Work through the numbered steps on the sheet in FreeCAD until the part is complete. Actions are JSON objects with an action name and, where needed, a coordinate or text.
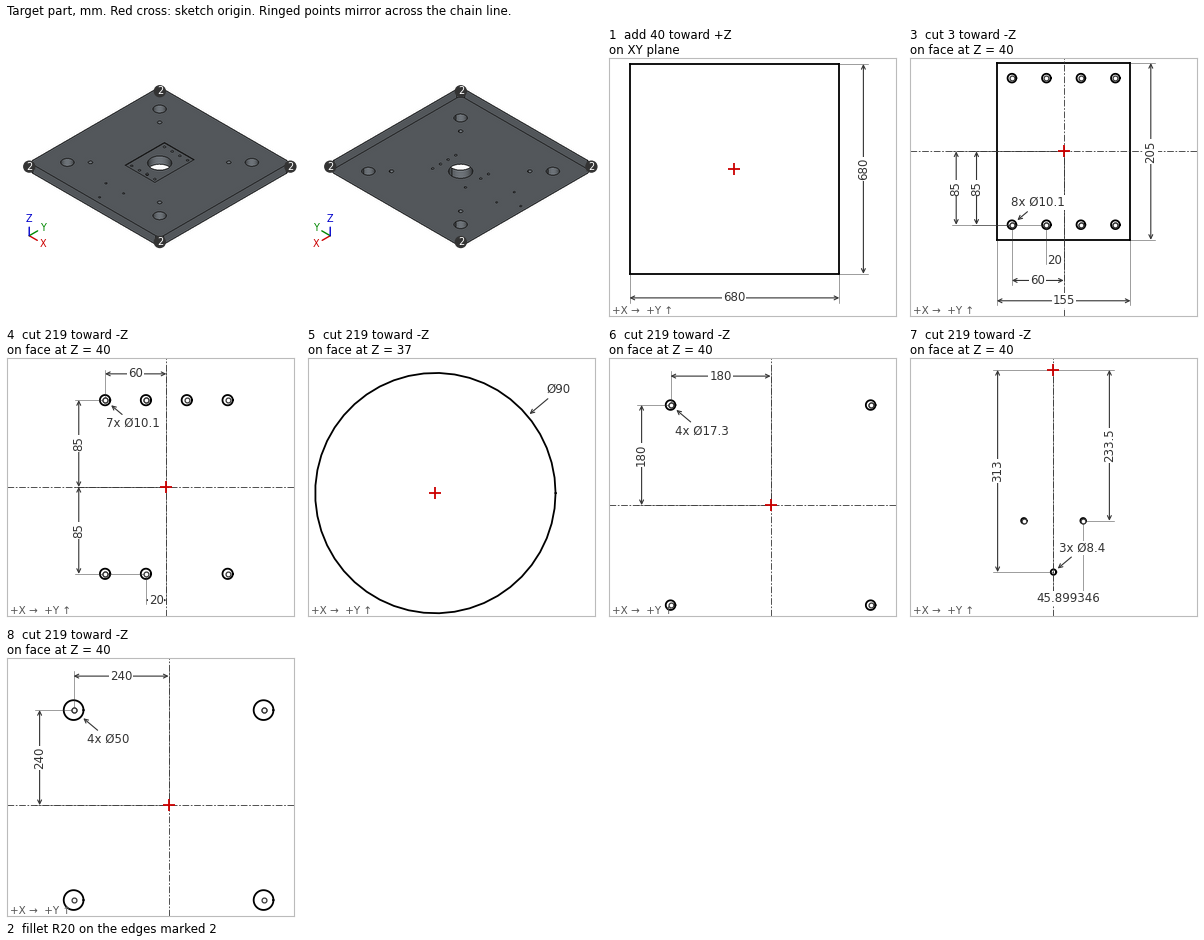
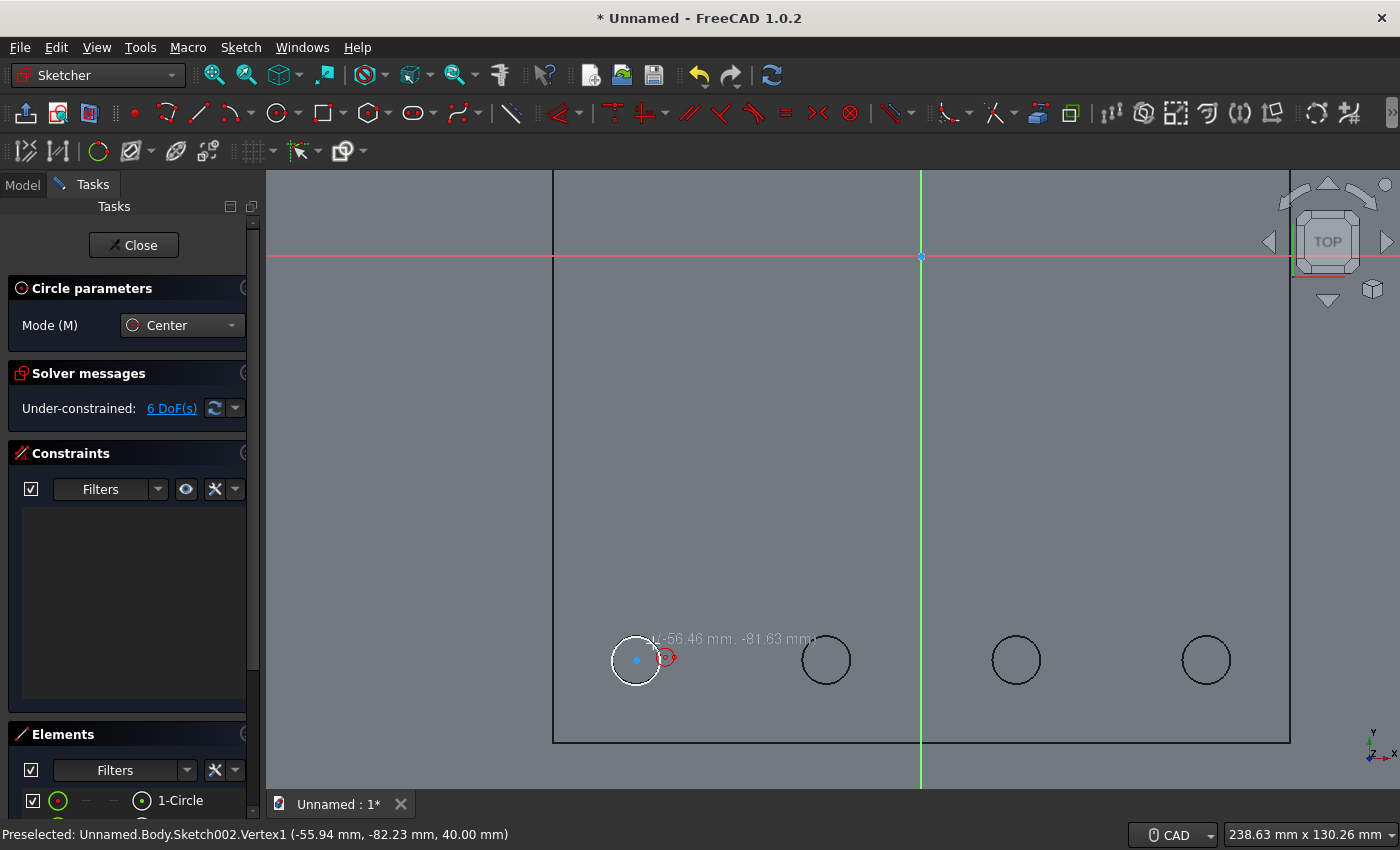
{"action": "left_click", "coordinate": [826, 660]}
{"action": "left_click", "coordinate": [843, 643]}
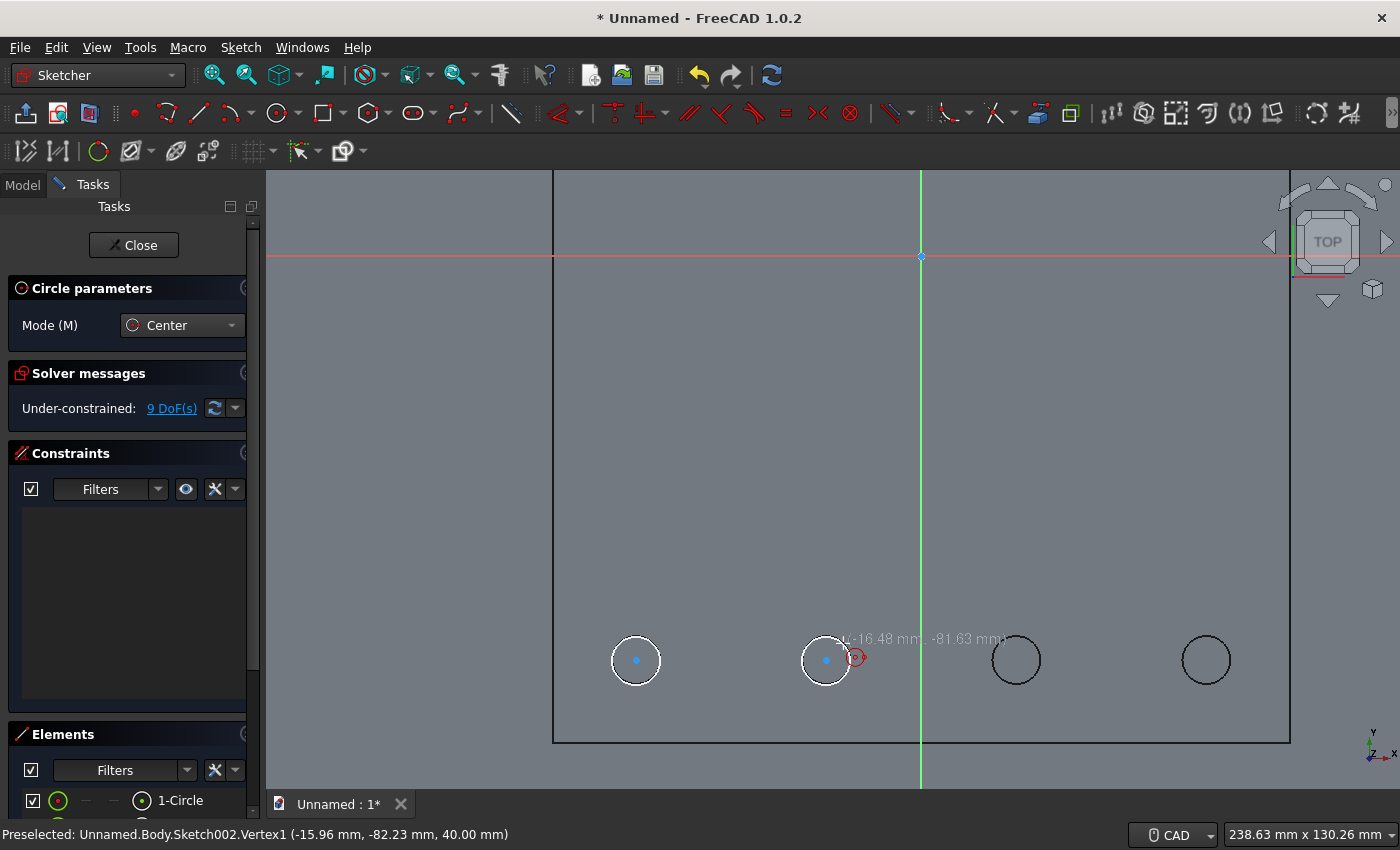
{"action": "left_click", "coordinate": [1206, 660]}
{"action": "left_click", "coordinate": [1223, 643]}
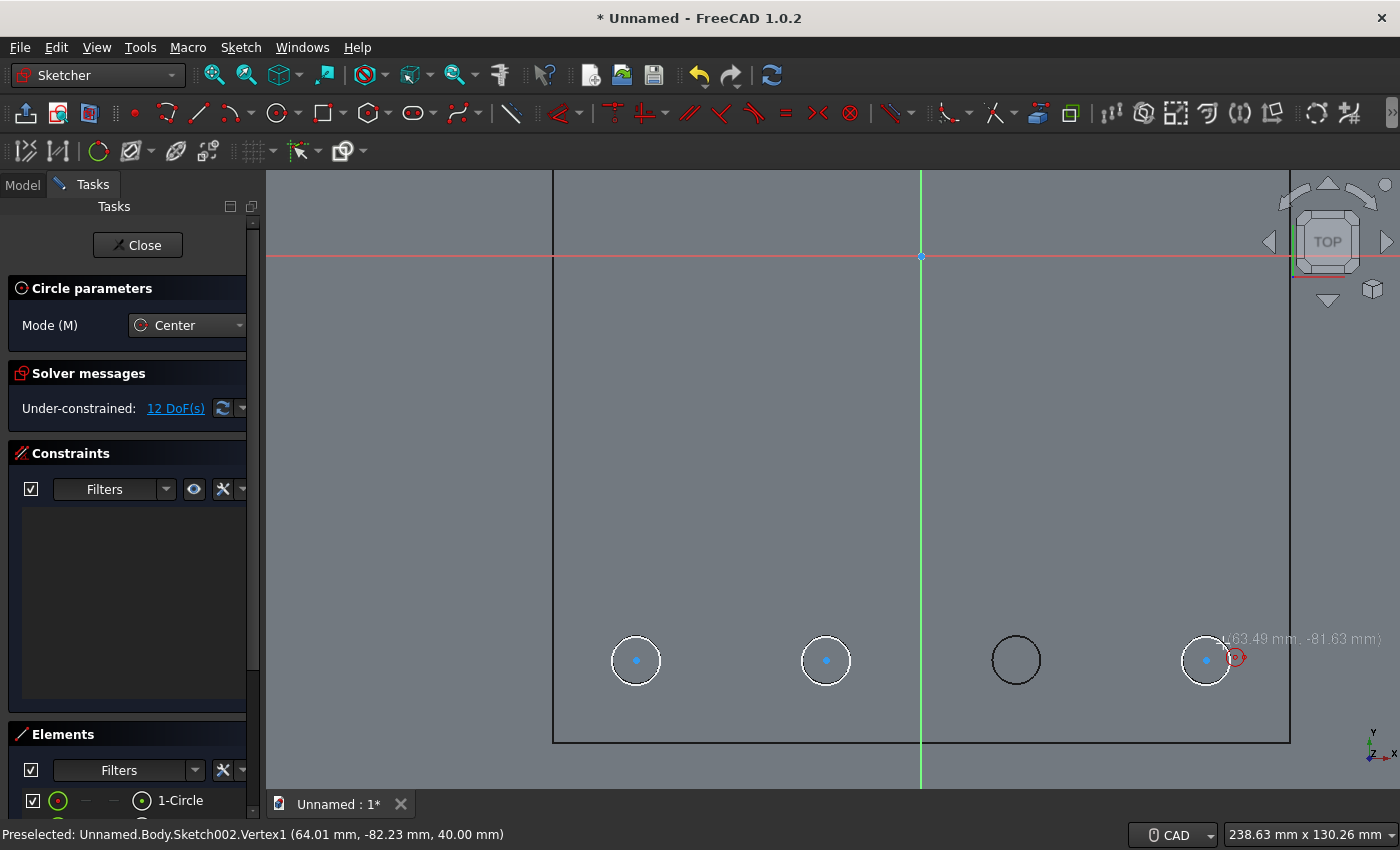
{"action": "scroll", "coordinate": [637, 662], "scroll_direction": "down", "scroll_amount": 4}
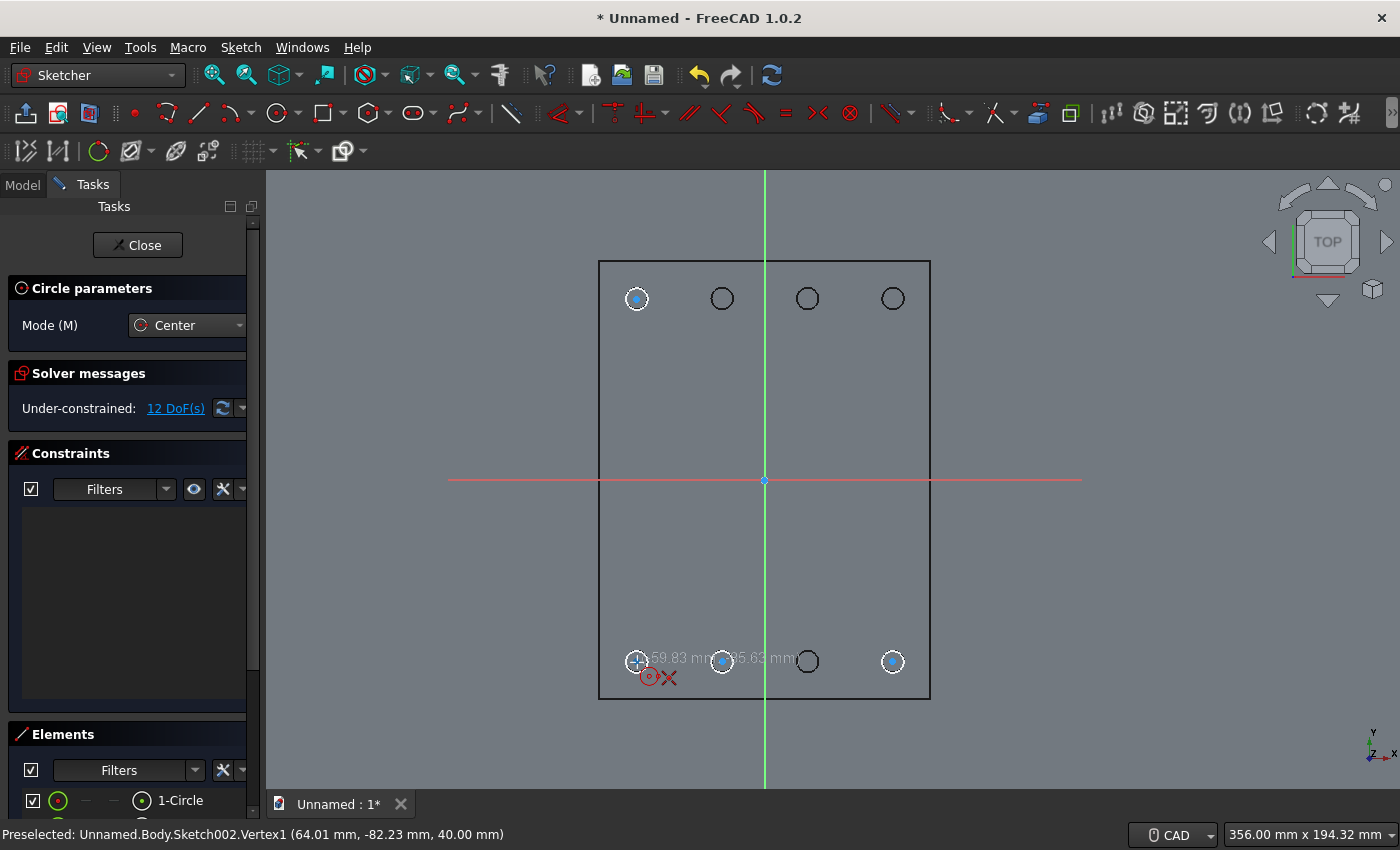
{"action": "scroll", "coordinate": [893, 299], "scroll_direction": "up", "scroll_amount": 4}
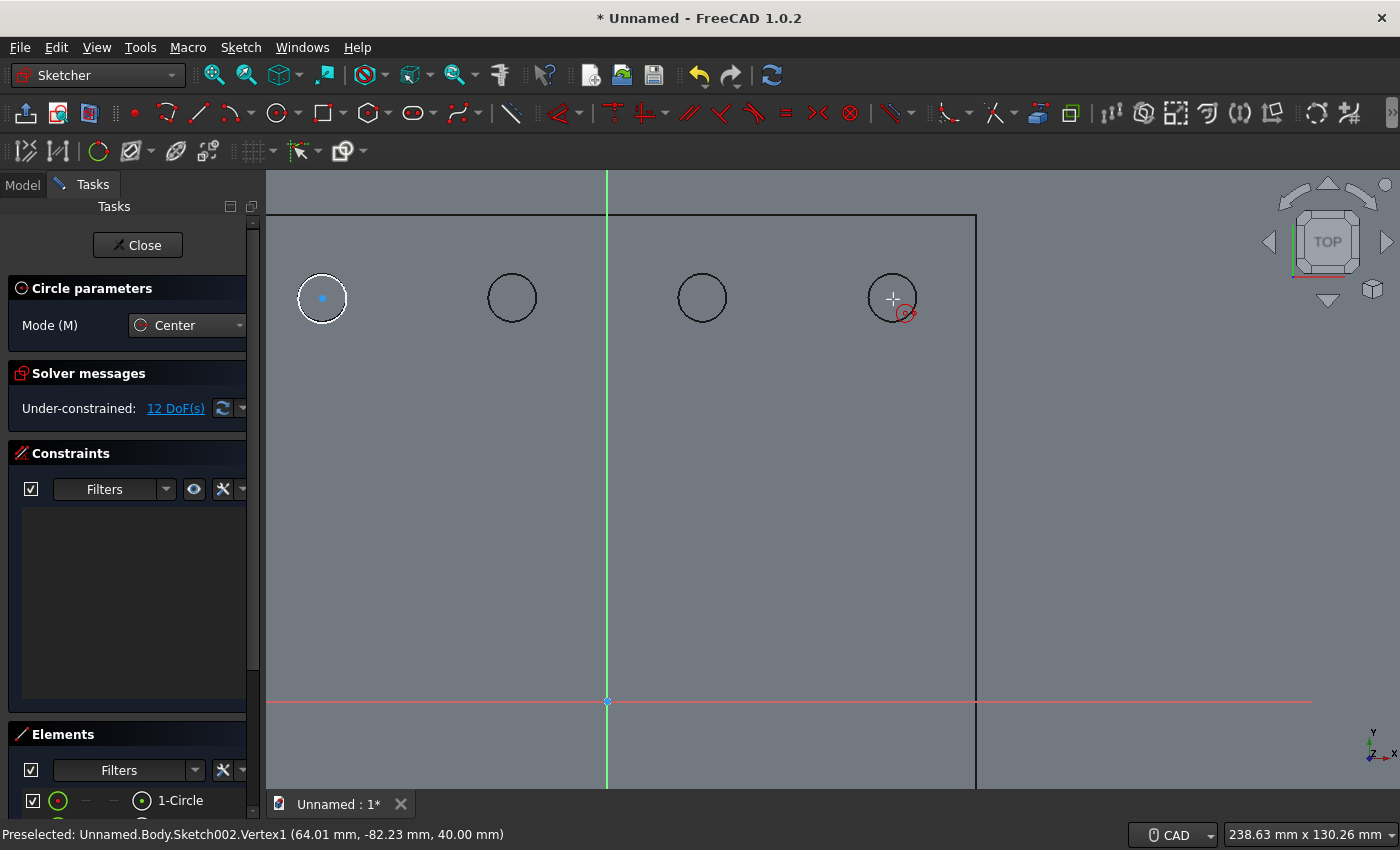
{"action": "left_click", "coordinate": [892, 298]}
{"action": "left_click", "coordinate": [909, 281]}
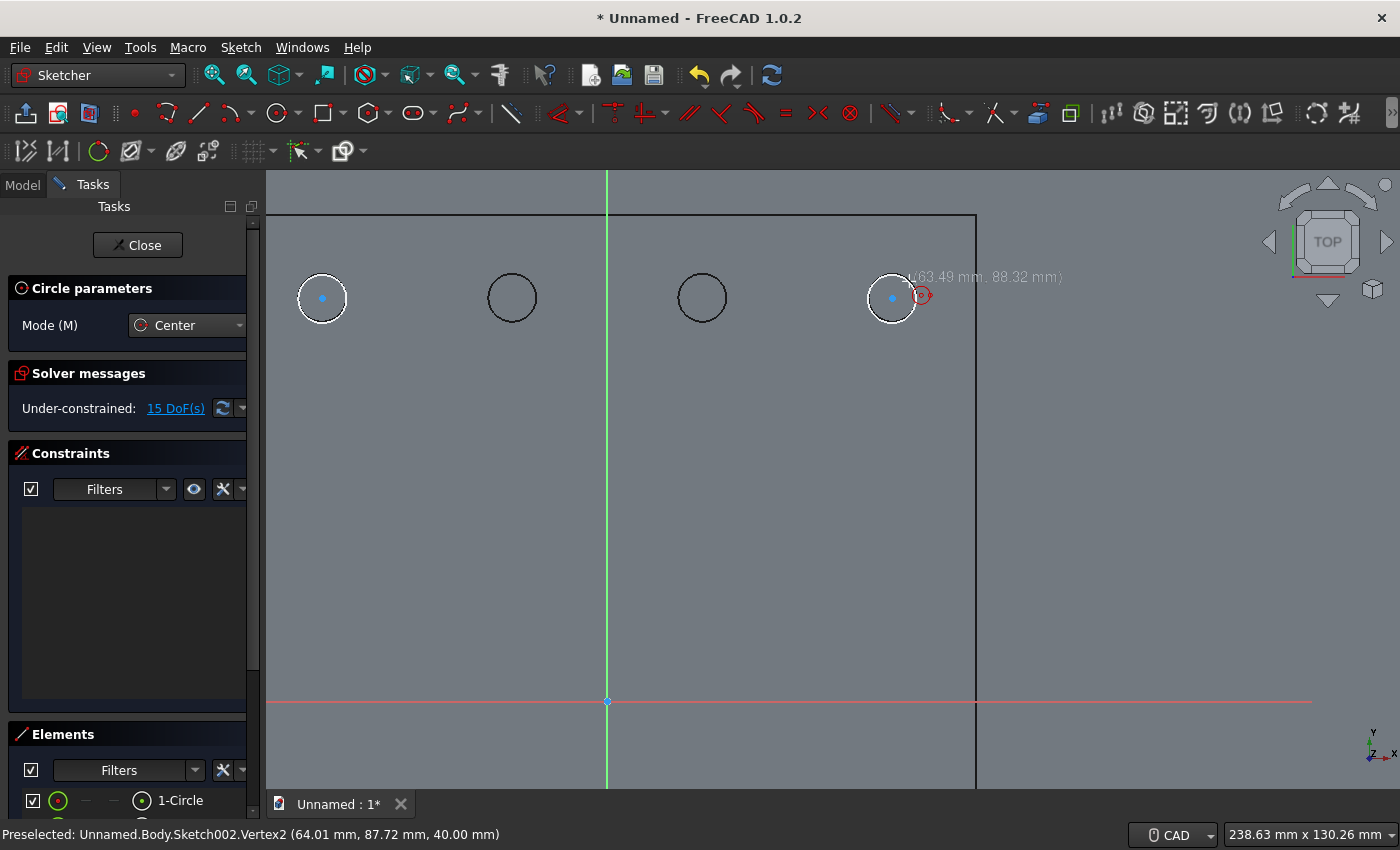
{"action": "left_click", "coordinate": [702, 298]}
{"action": "left_click", "coordinate": [719, 281]}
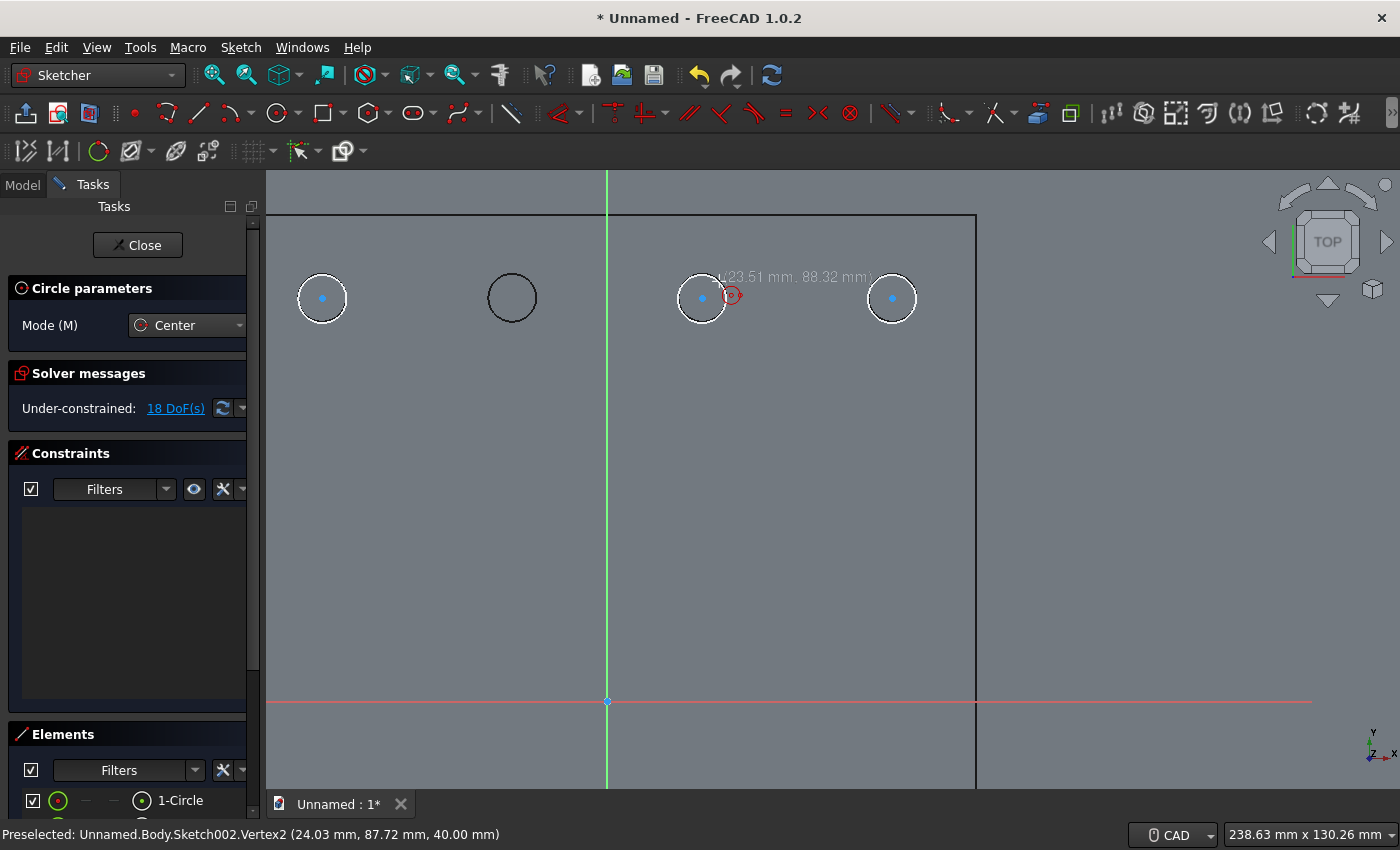
{"action": "left_click", "coordinate": [512, 298]}
{"action": "left_click", "coordinate": [529, 281]}
{"action": "key", "text": "Escape"}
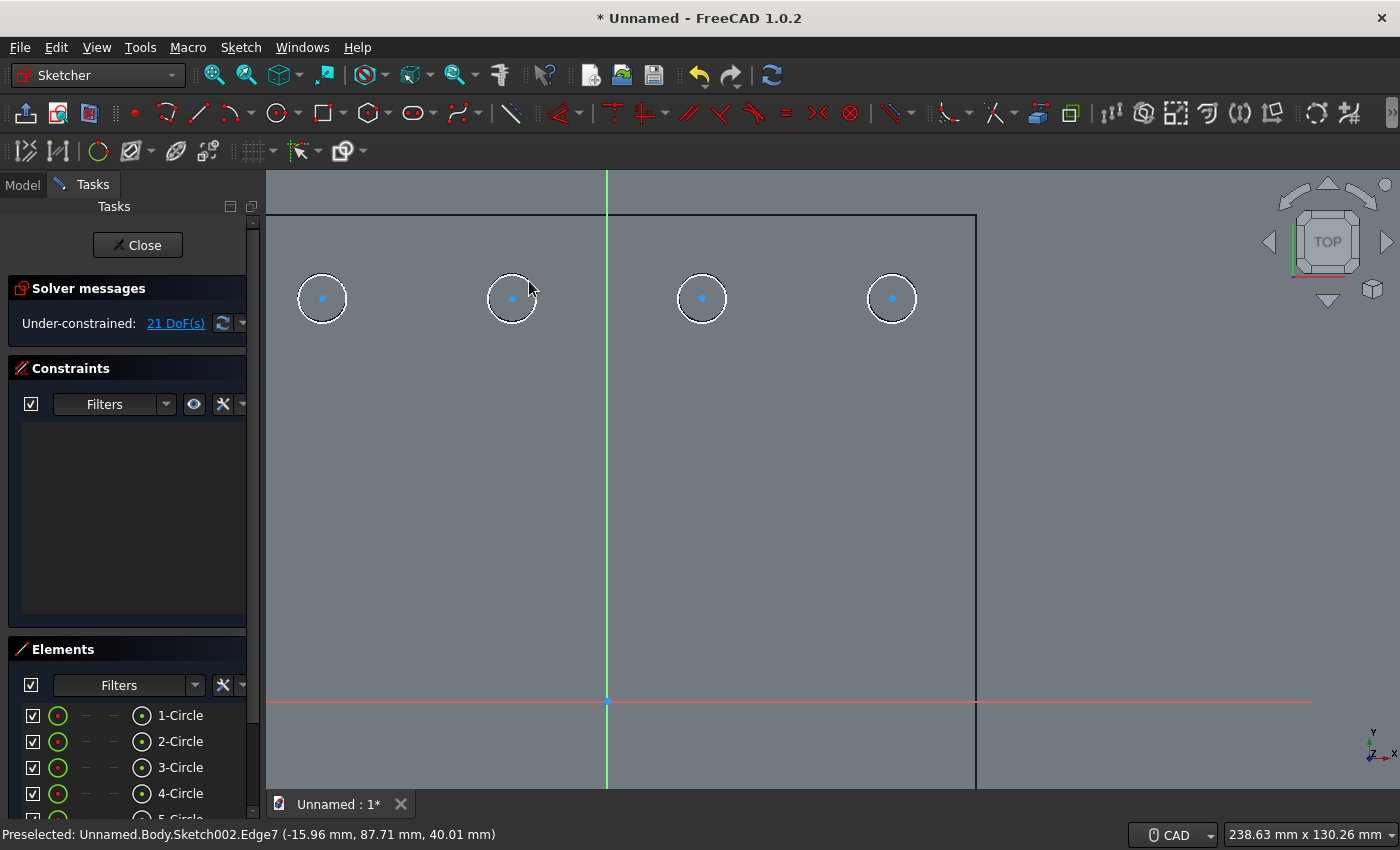
{"action": "left_click", "coordinate": [339, 282]}